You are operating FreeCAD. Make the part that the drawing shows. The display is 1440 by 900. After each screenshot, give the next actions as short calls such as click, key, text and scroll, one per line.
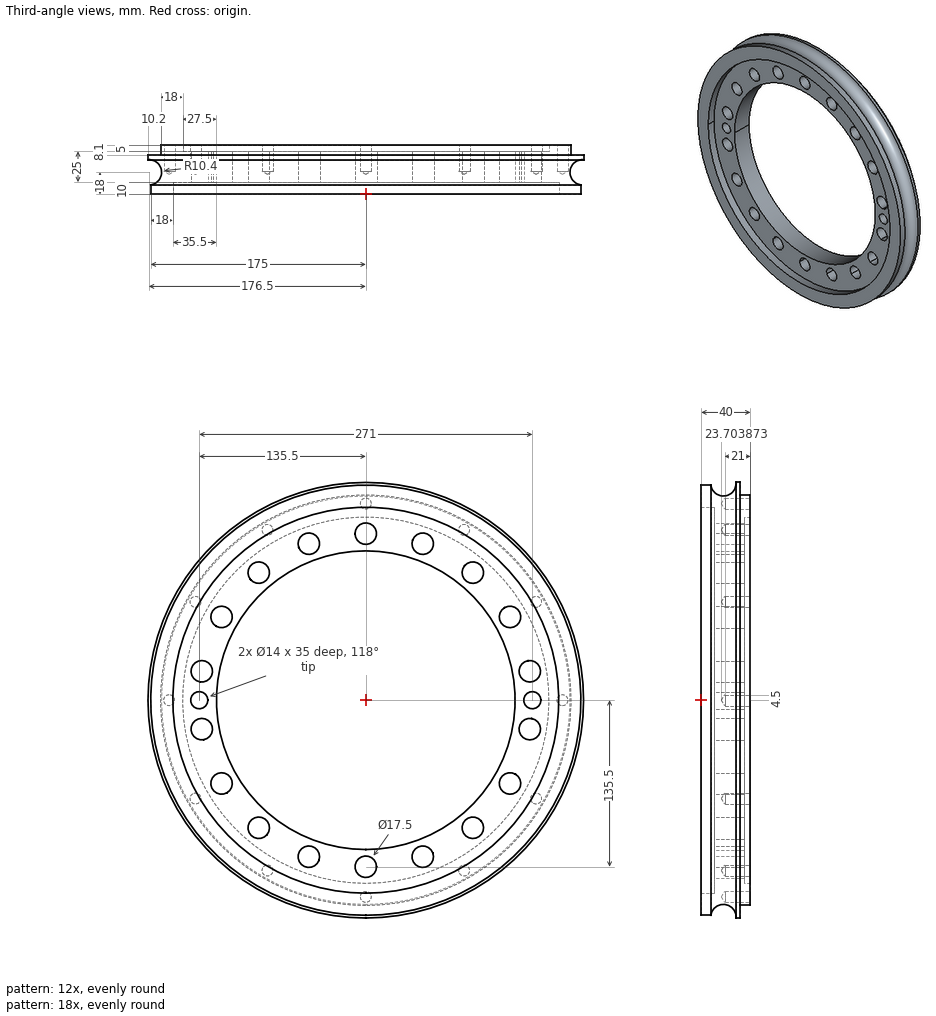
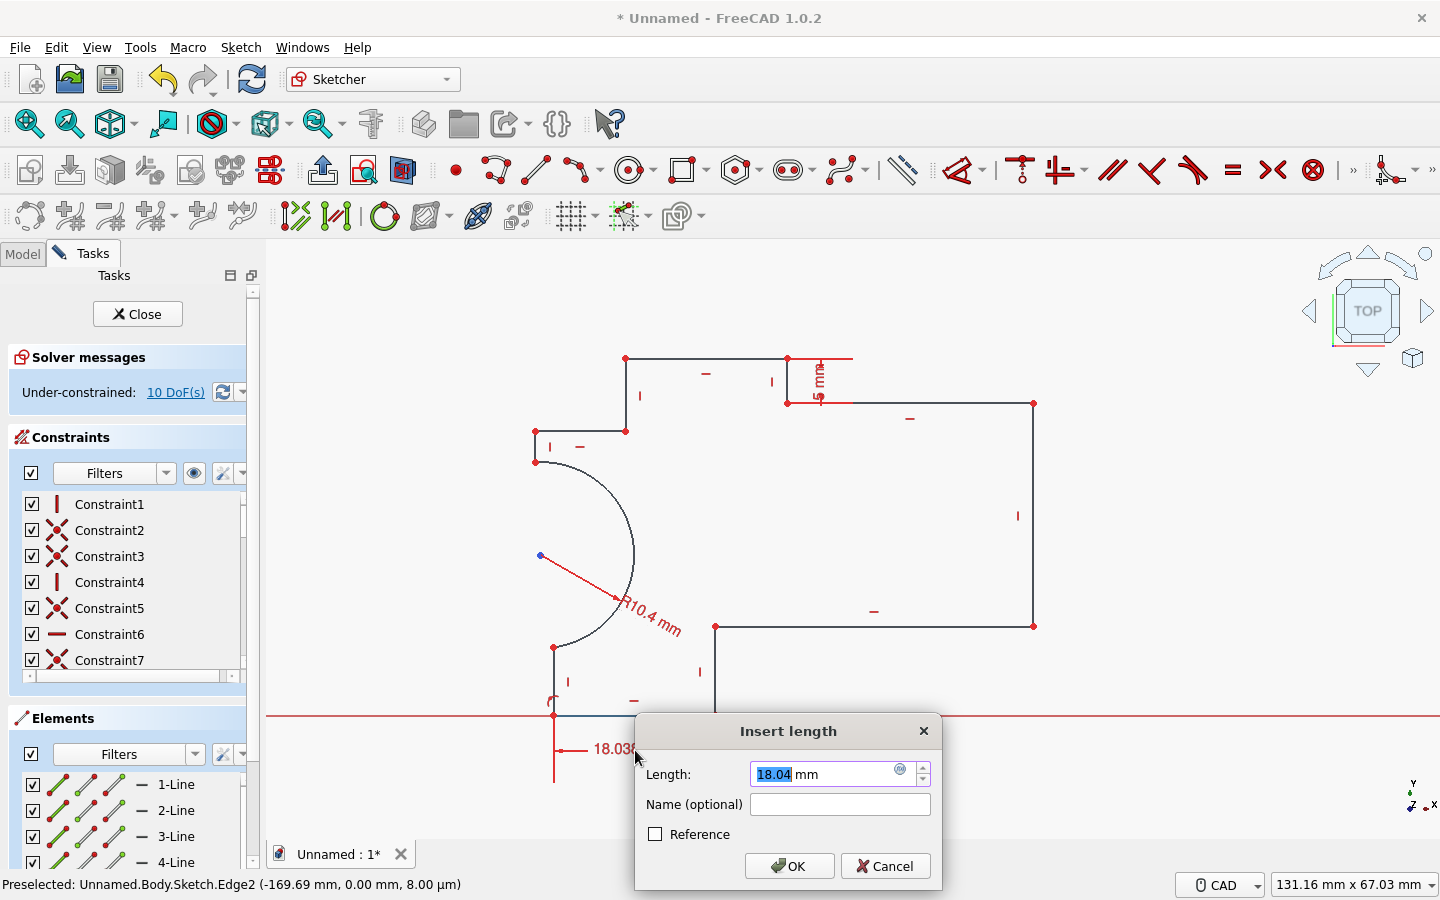
text(18)
key(Return)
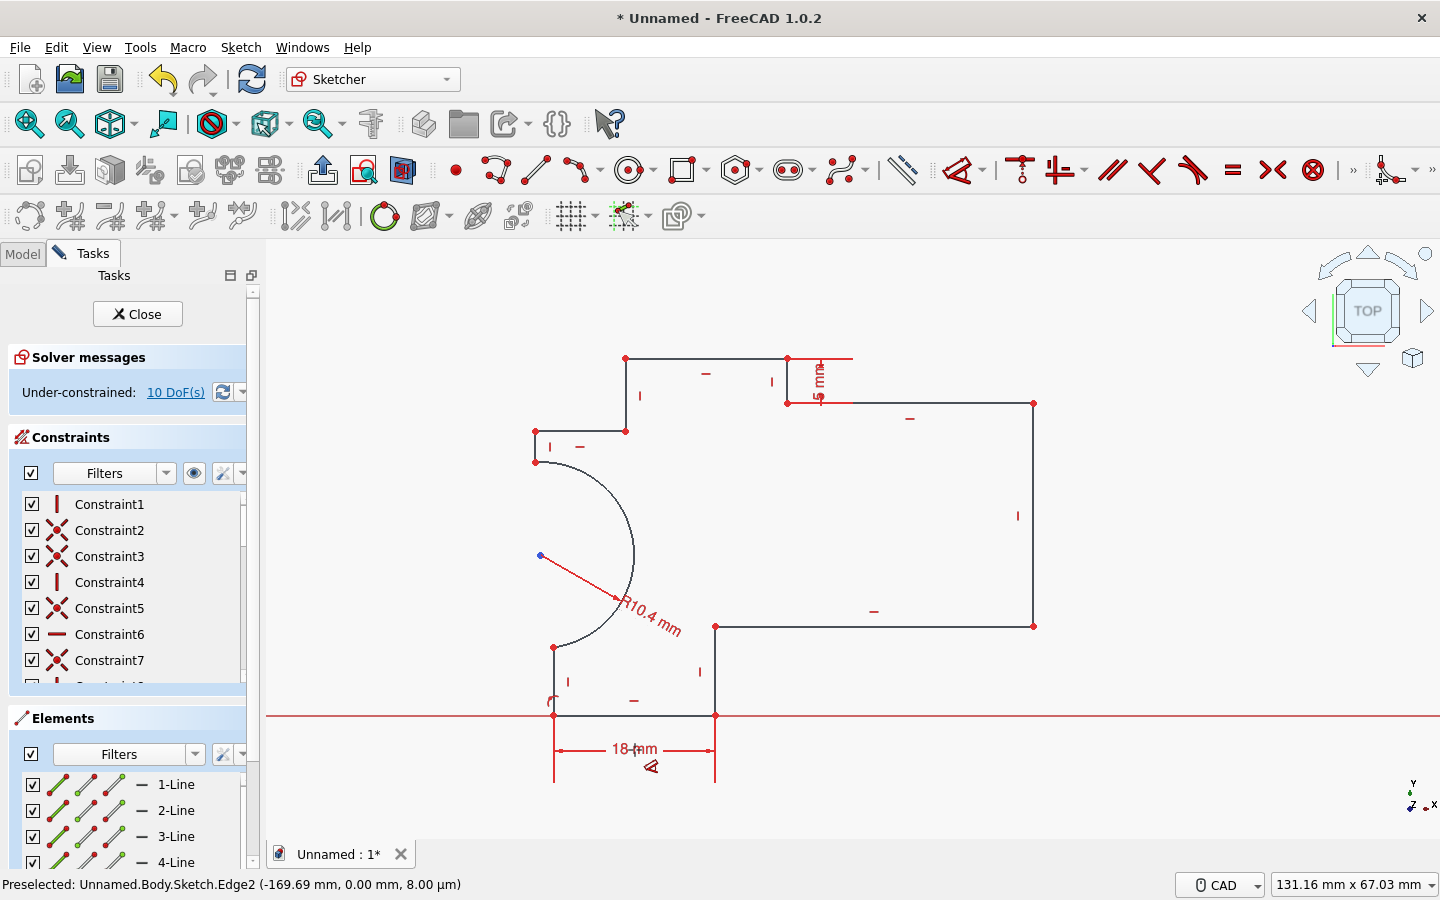
click(715, 689)
click(681, 671)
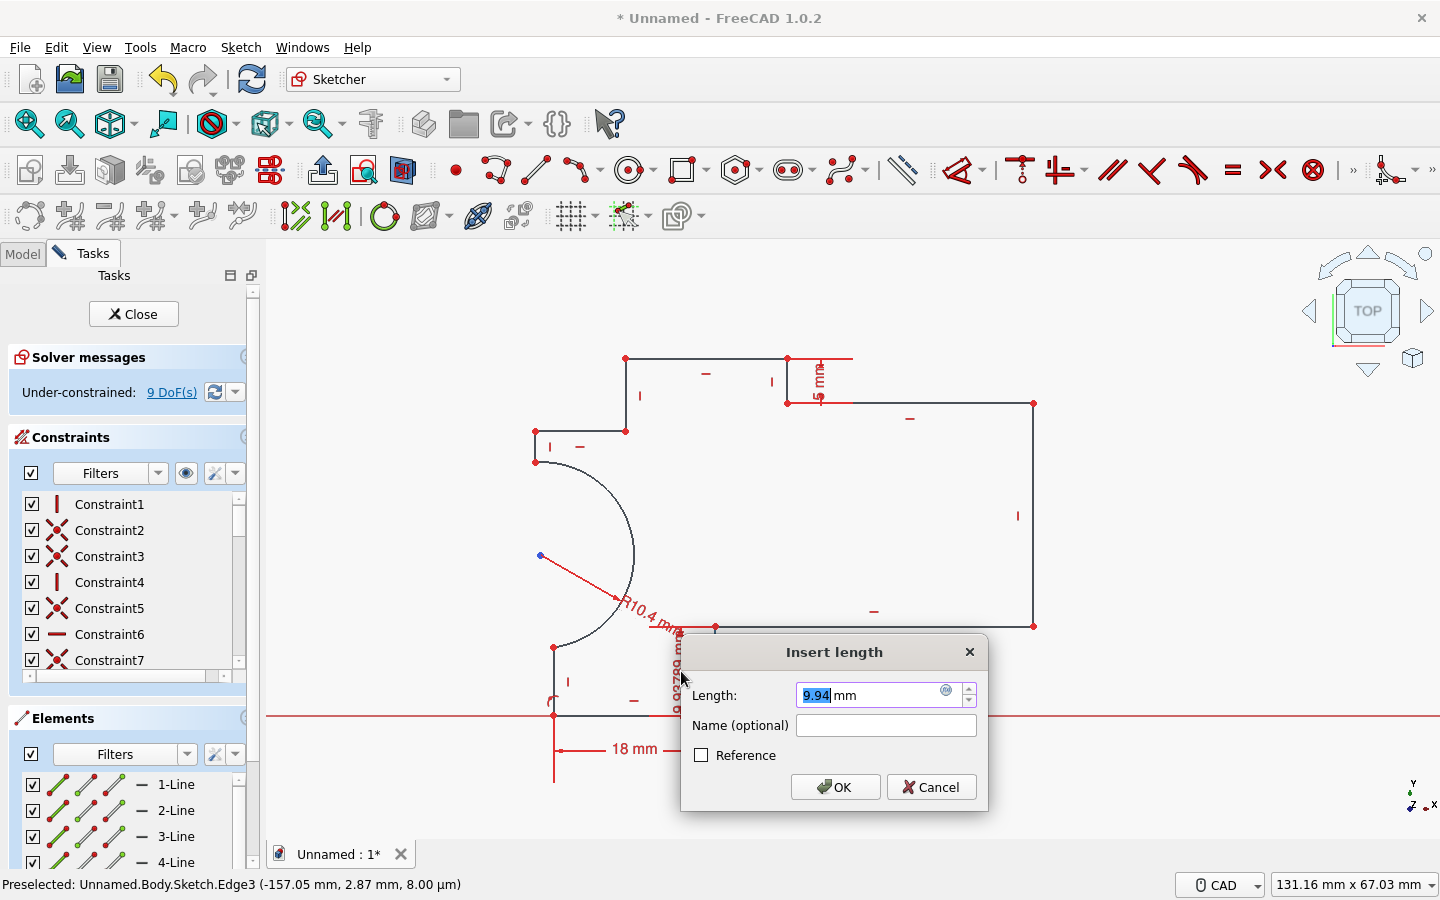
text(10)
key(Return)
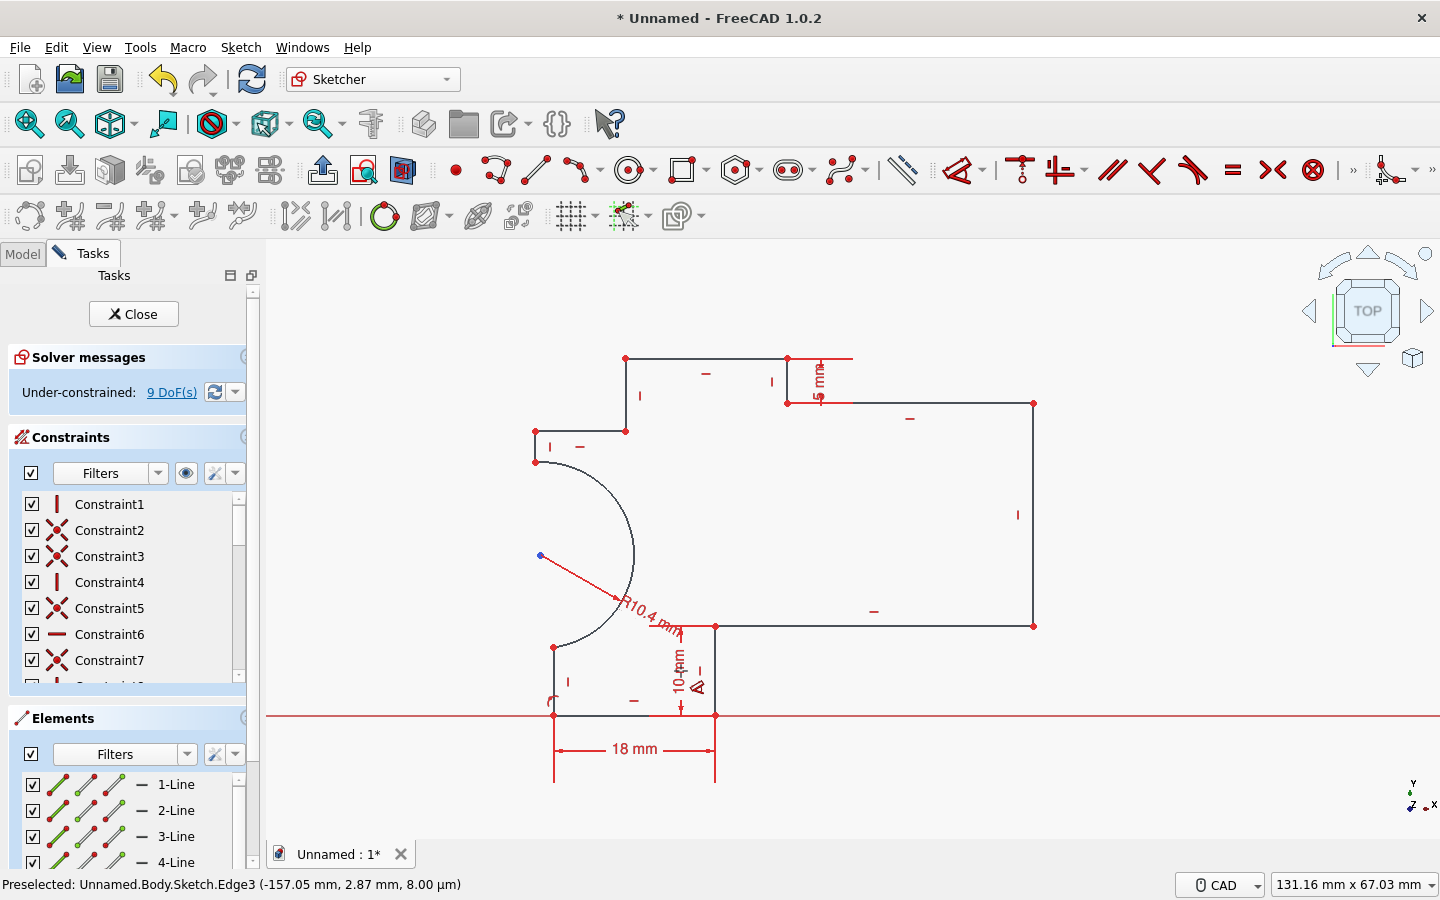
click(1033, 559)
click(1067, 515)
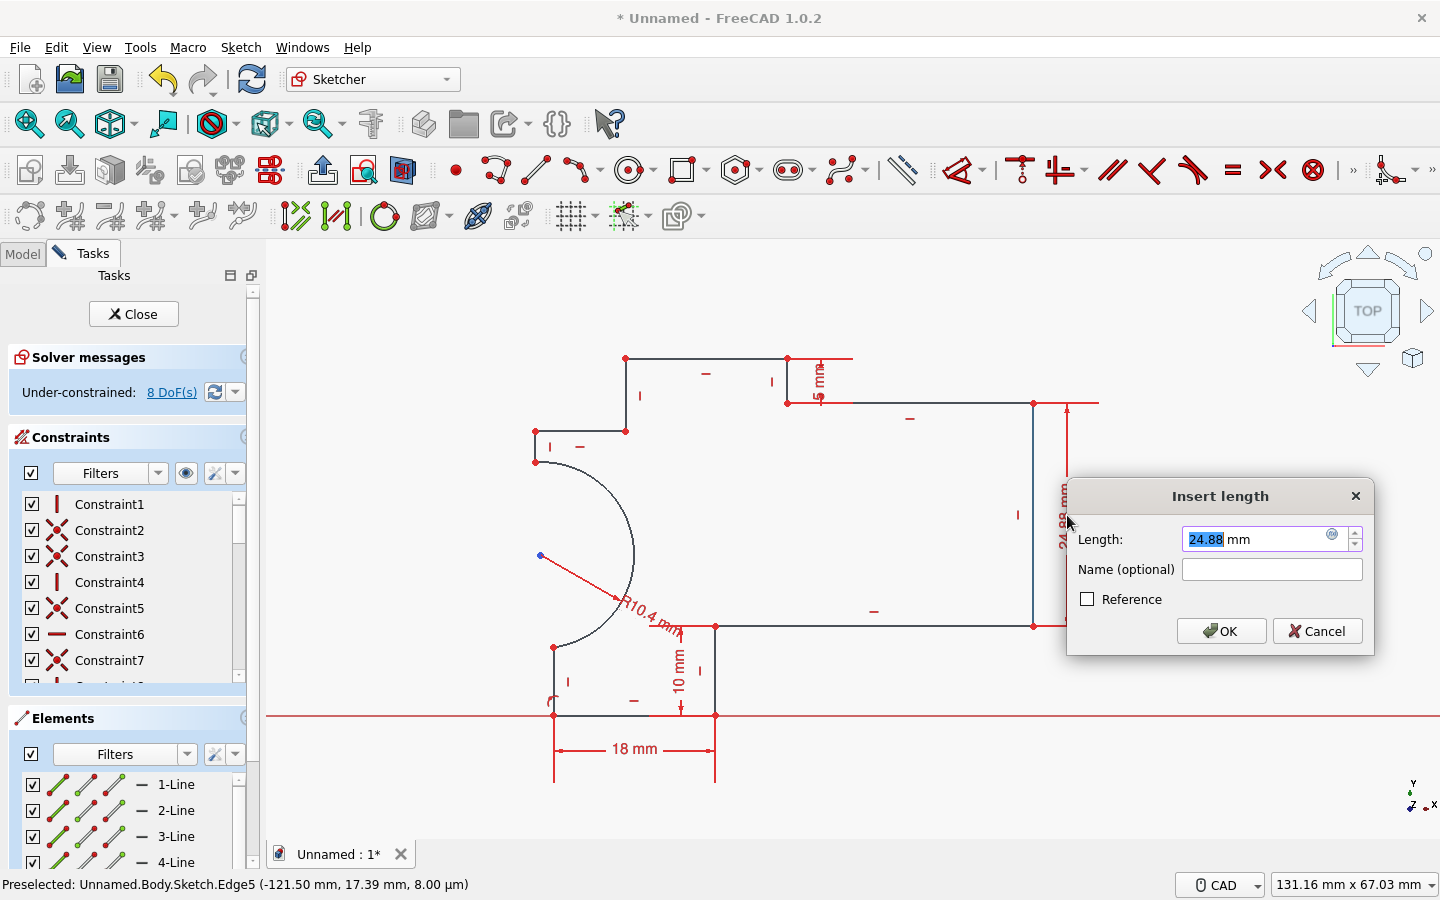
text(25)
key(Return)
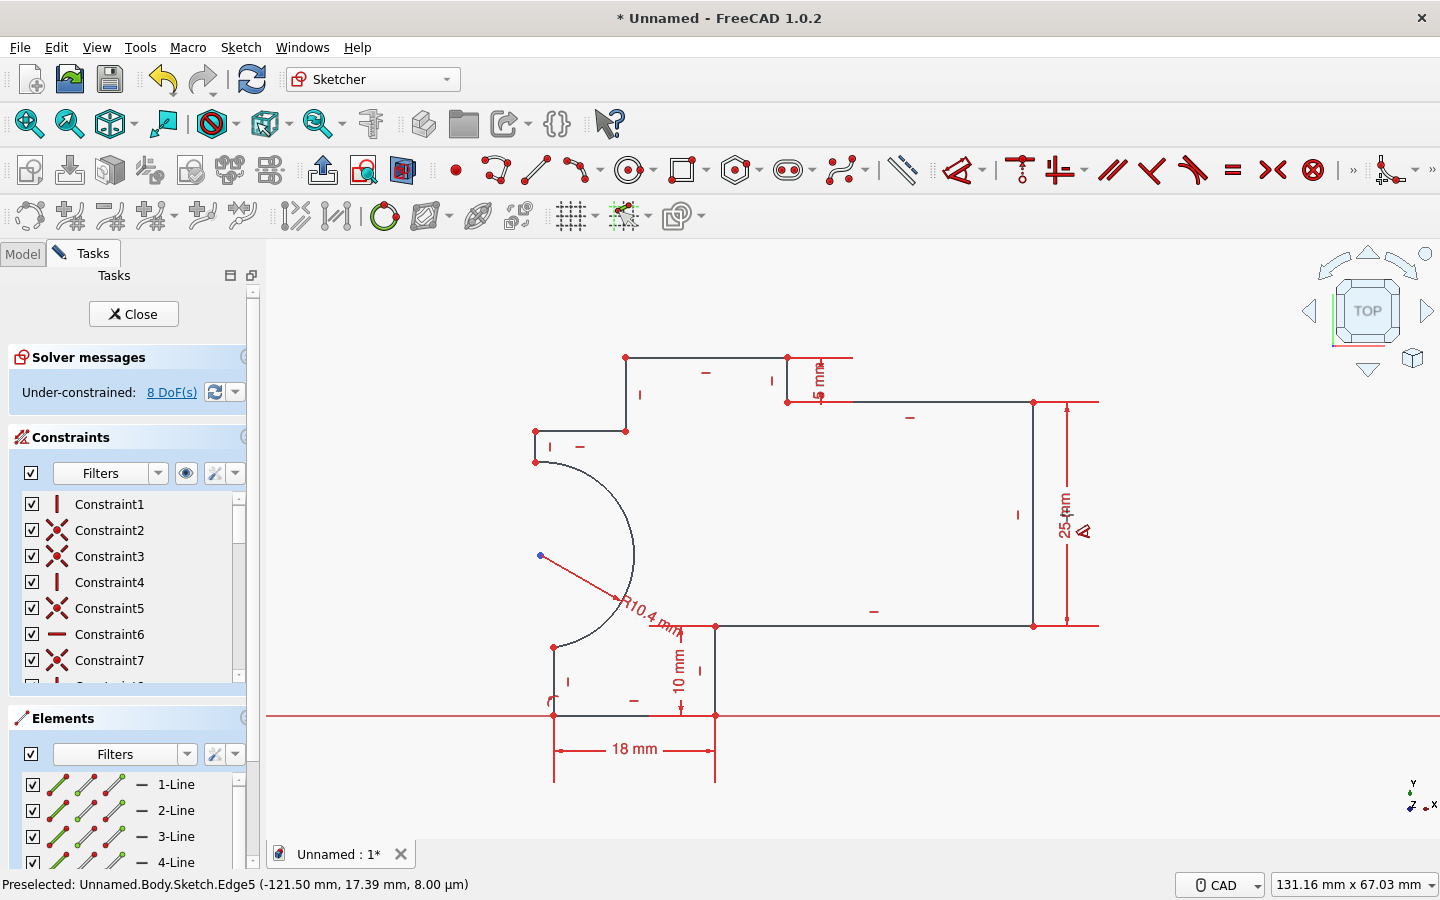
click(739, 358)
click(706, 324)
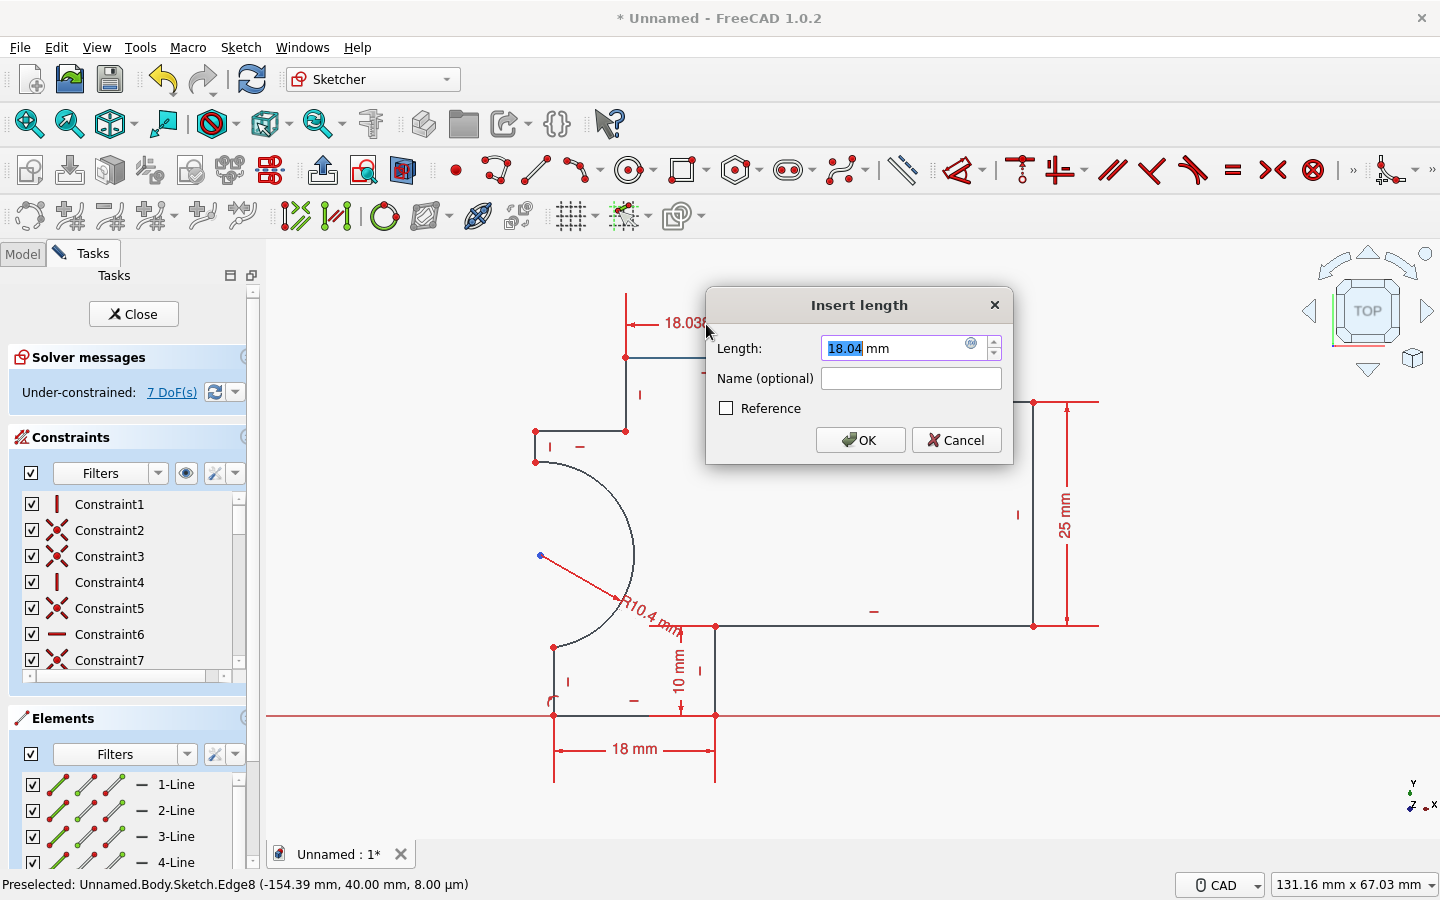
text(18)
key(Return)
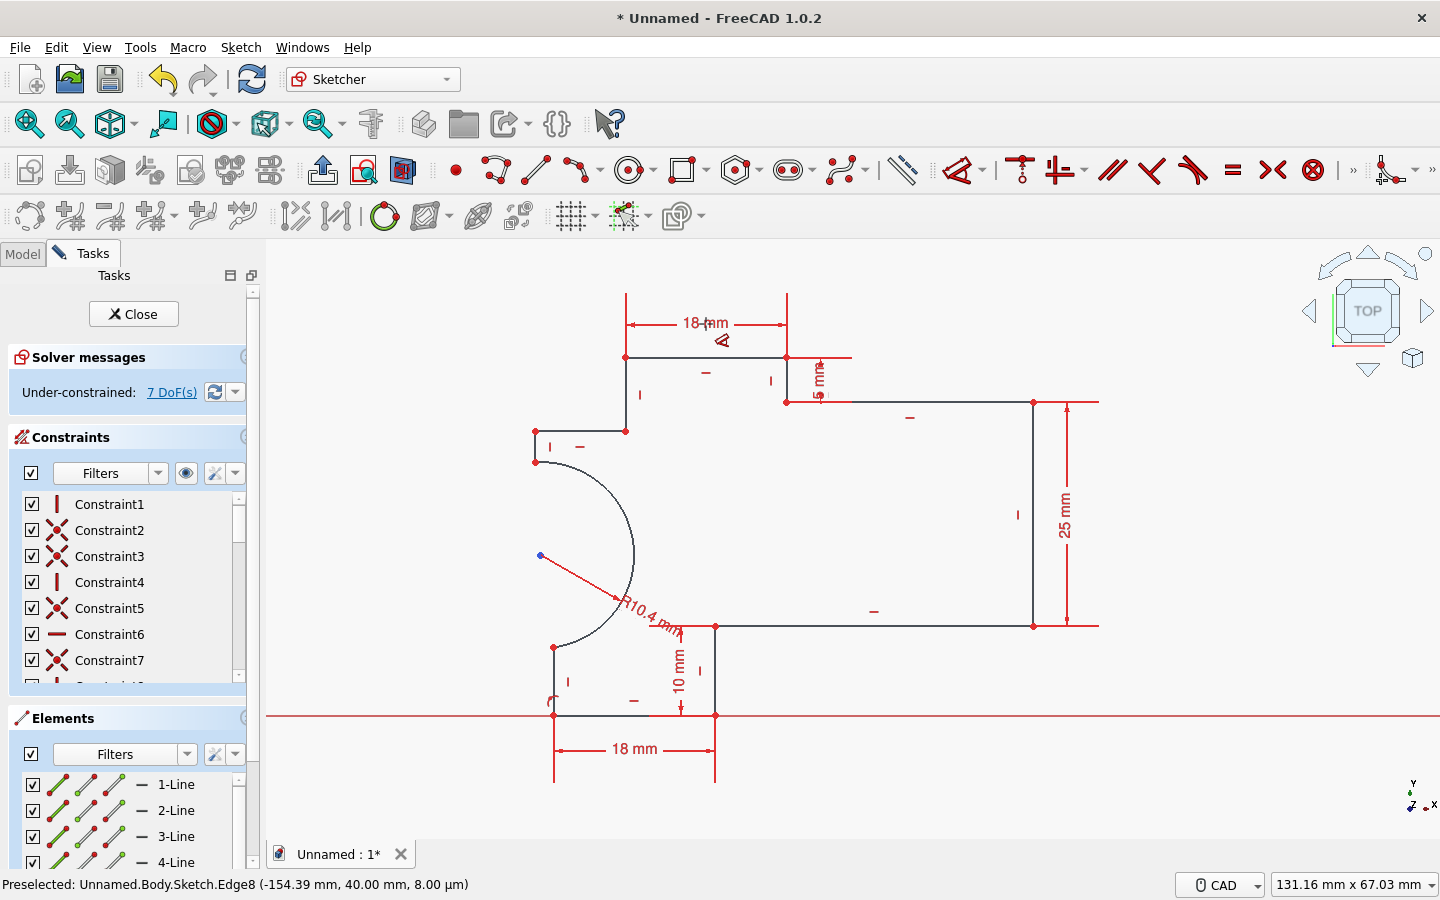
click(626, 380)
click(592, 394)